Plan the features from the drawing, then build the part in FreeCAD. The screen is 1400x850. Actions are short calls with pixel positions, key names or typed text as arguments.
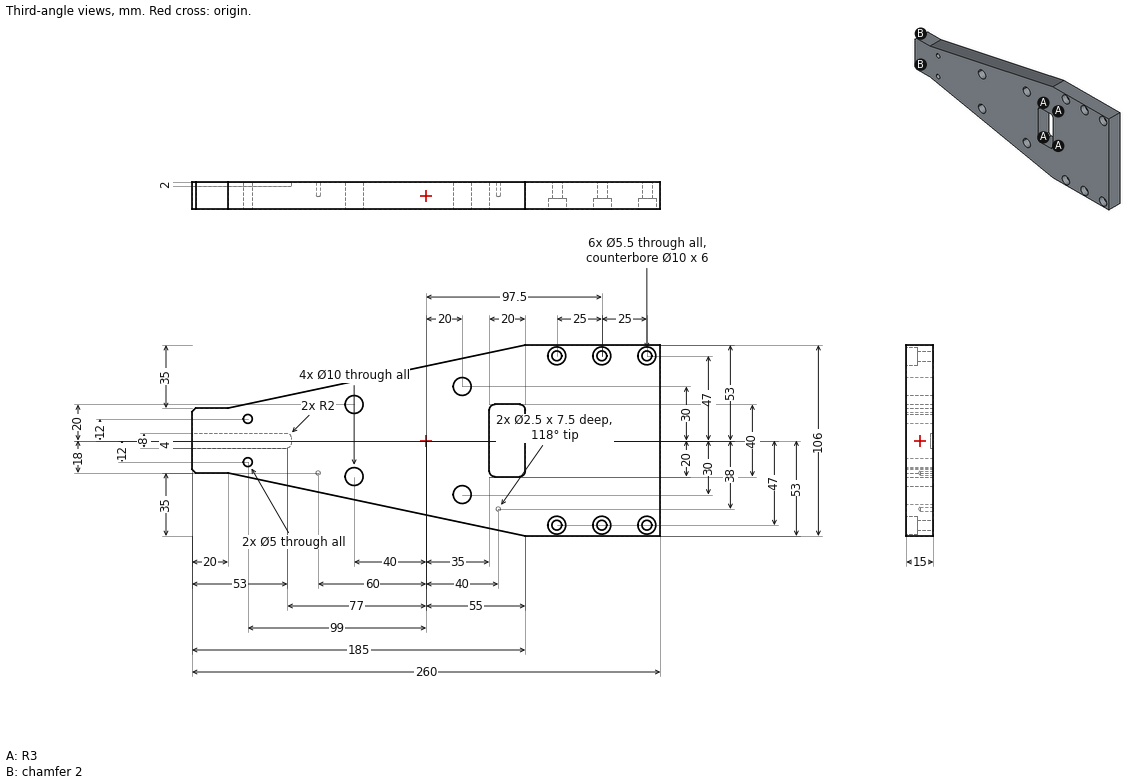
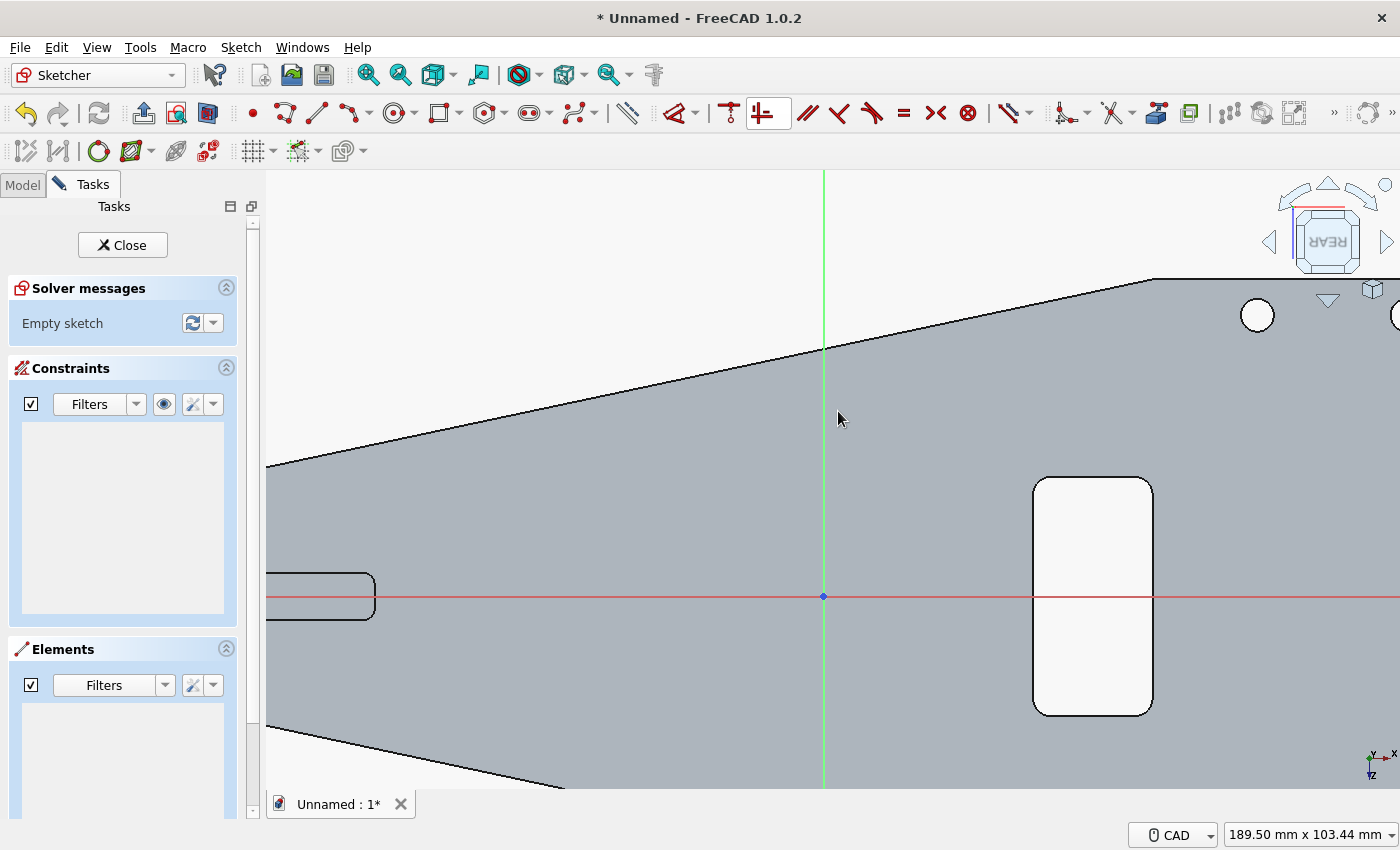
key(g)
key(c)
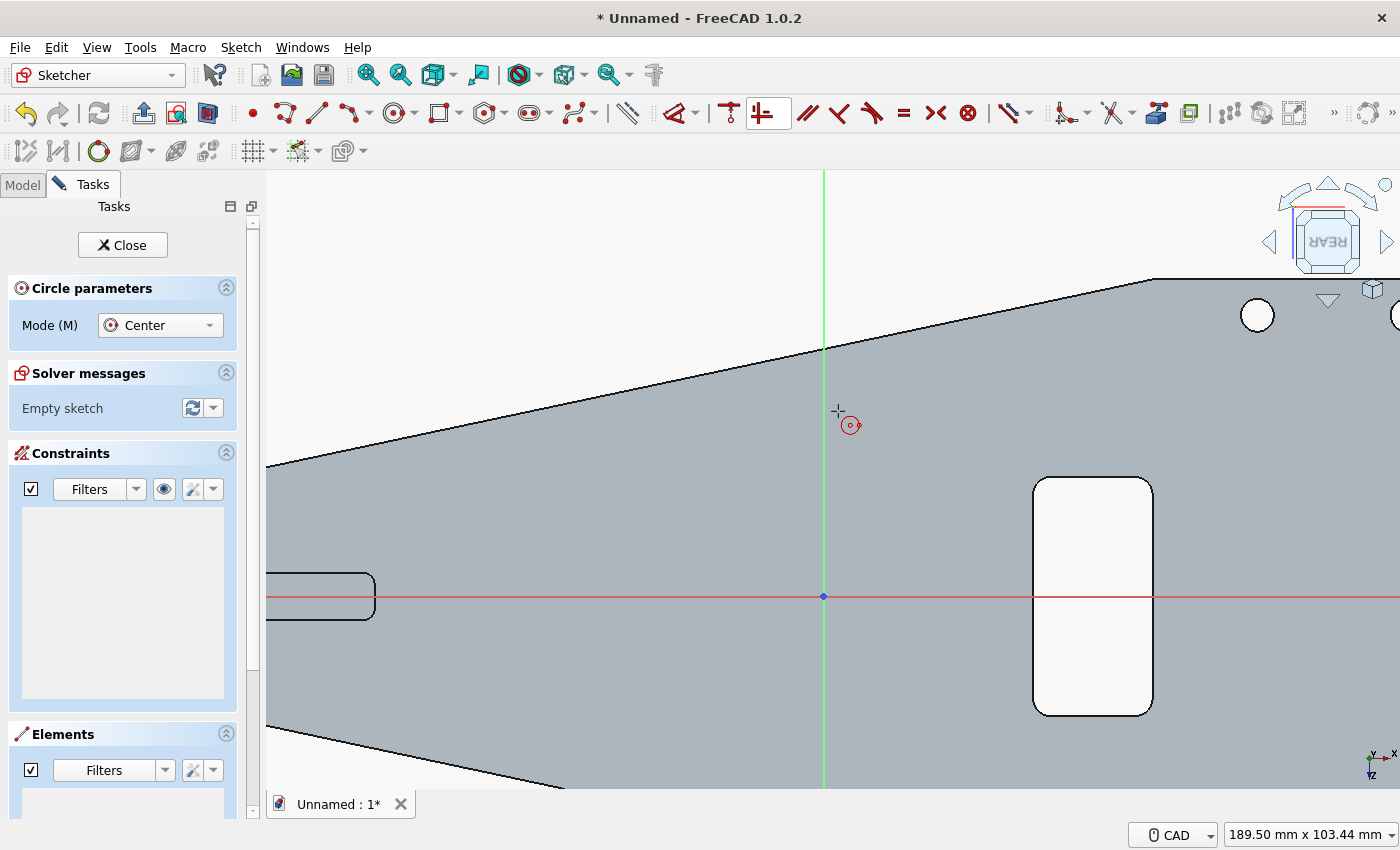
scroll(1063, 369, up, 6)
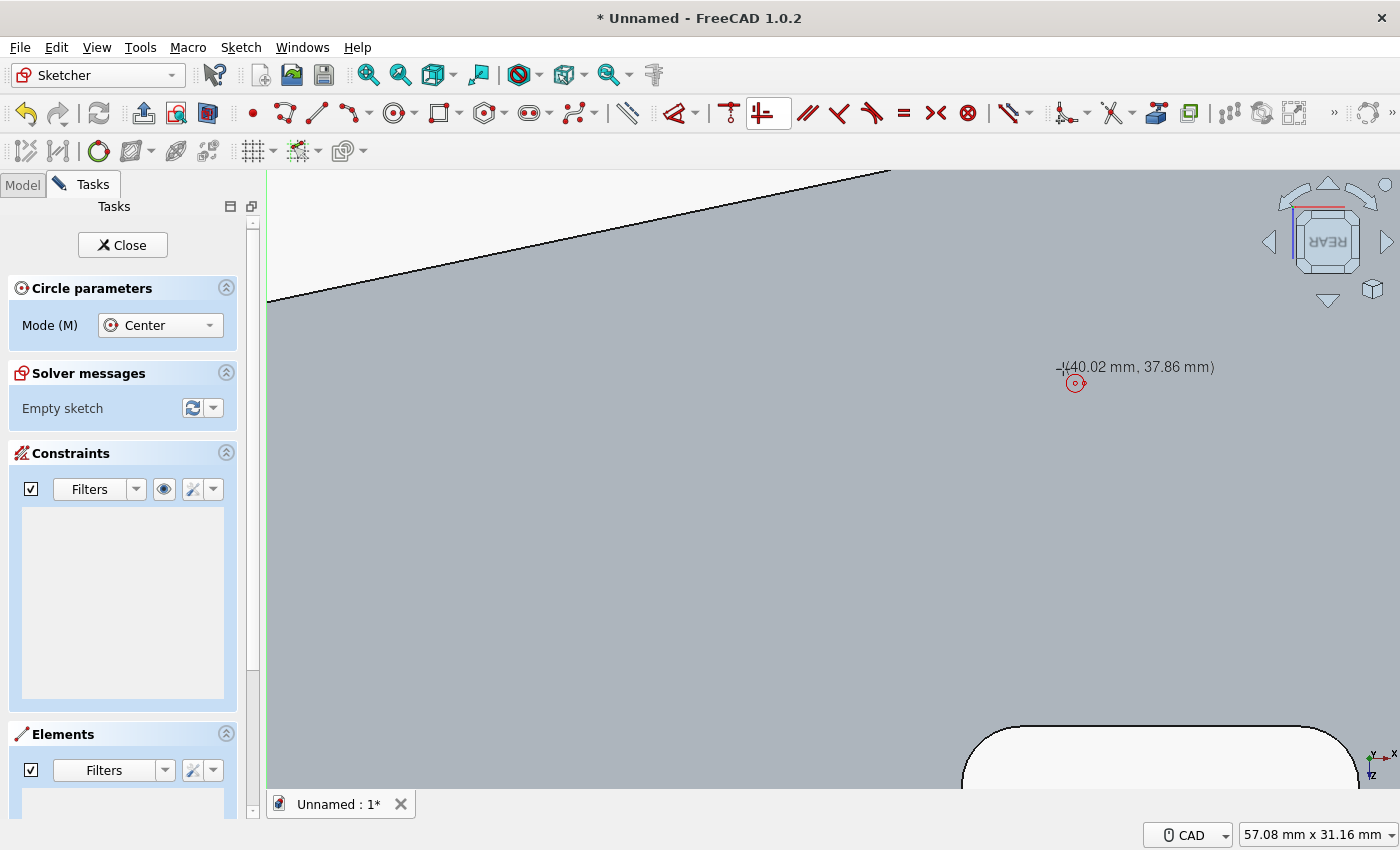
click(1061, 369)
click(1079, 351)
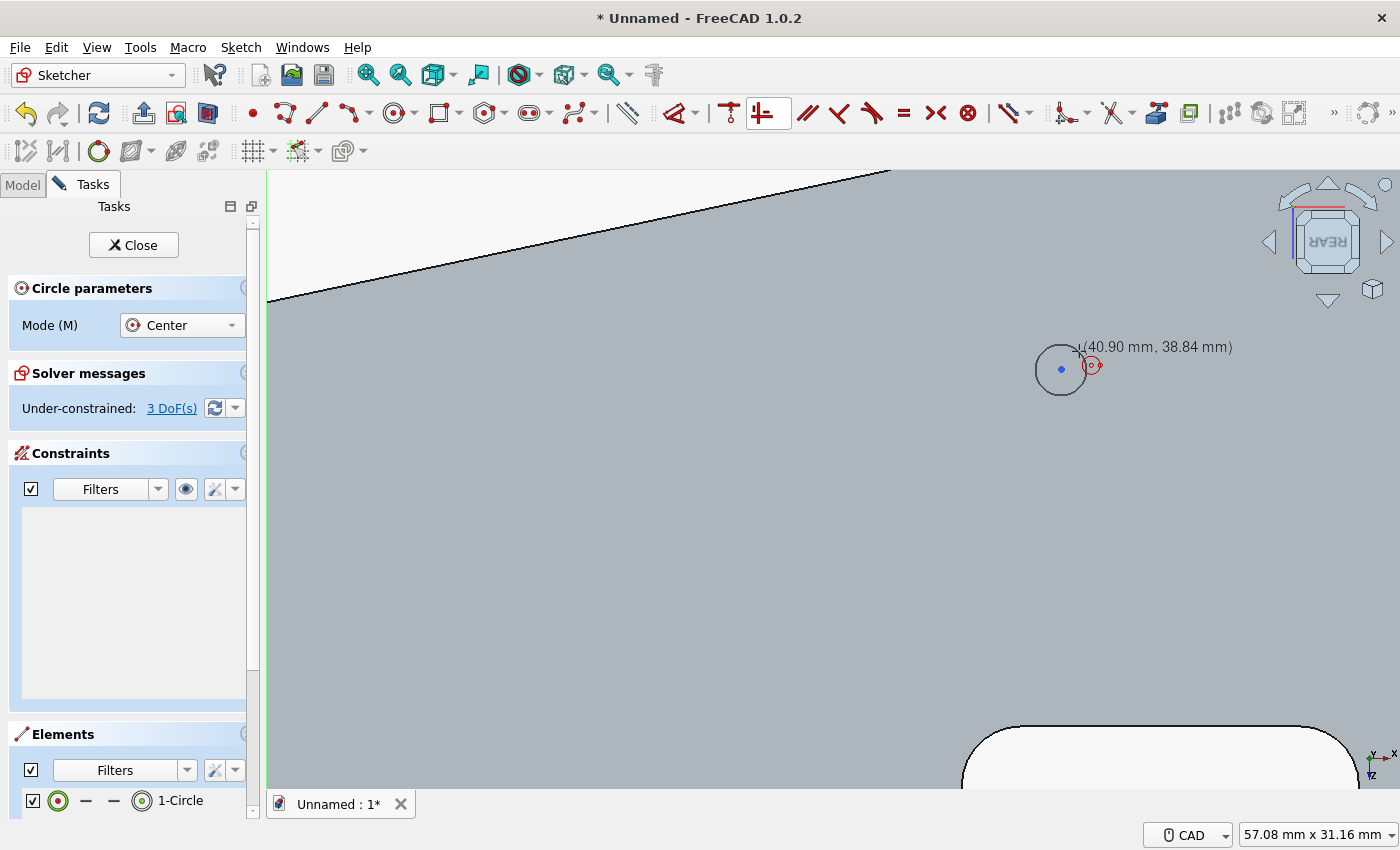
scroll(1065, 370, down, 6)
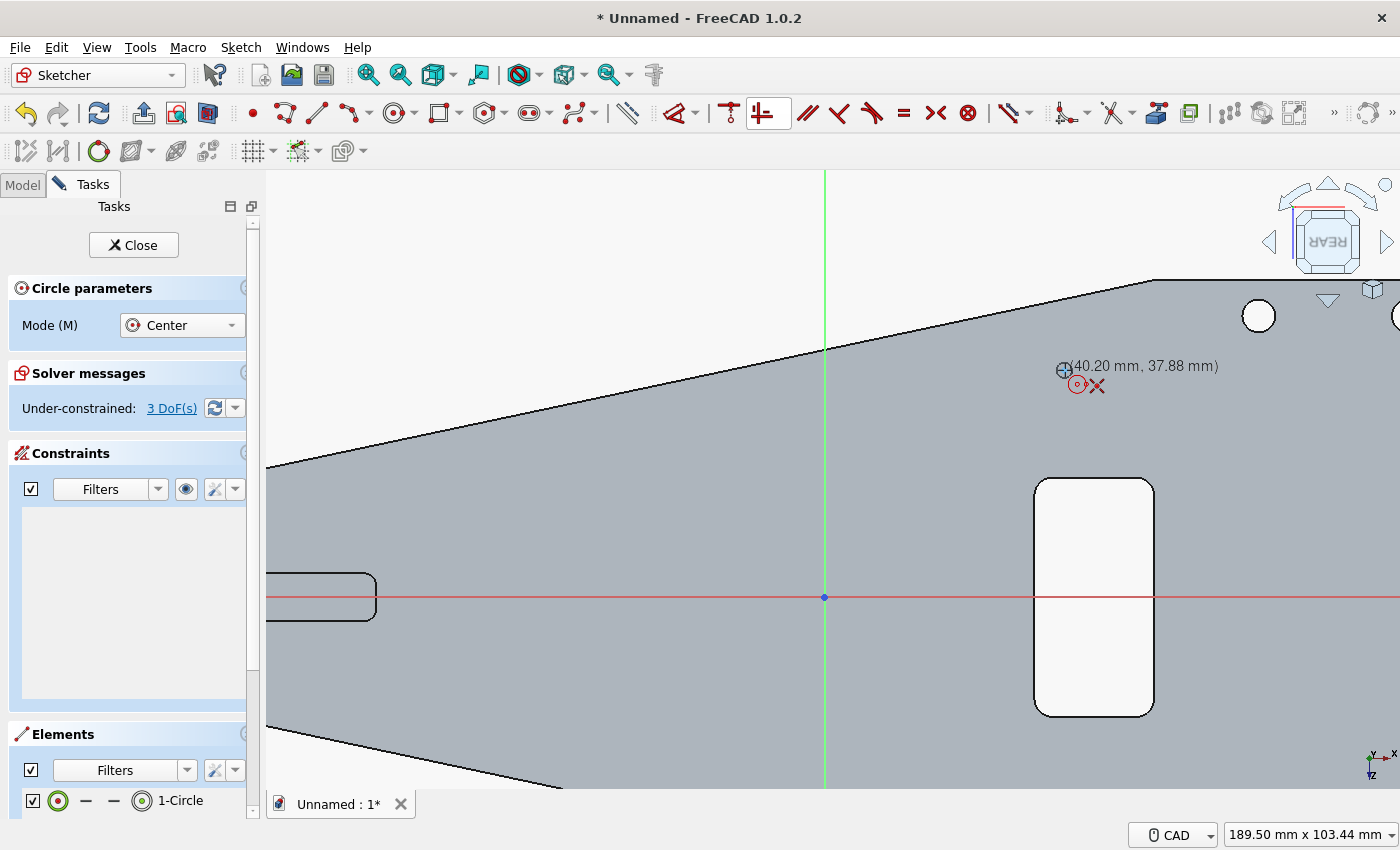
scroll(466, 490, up, 6)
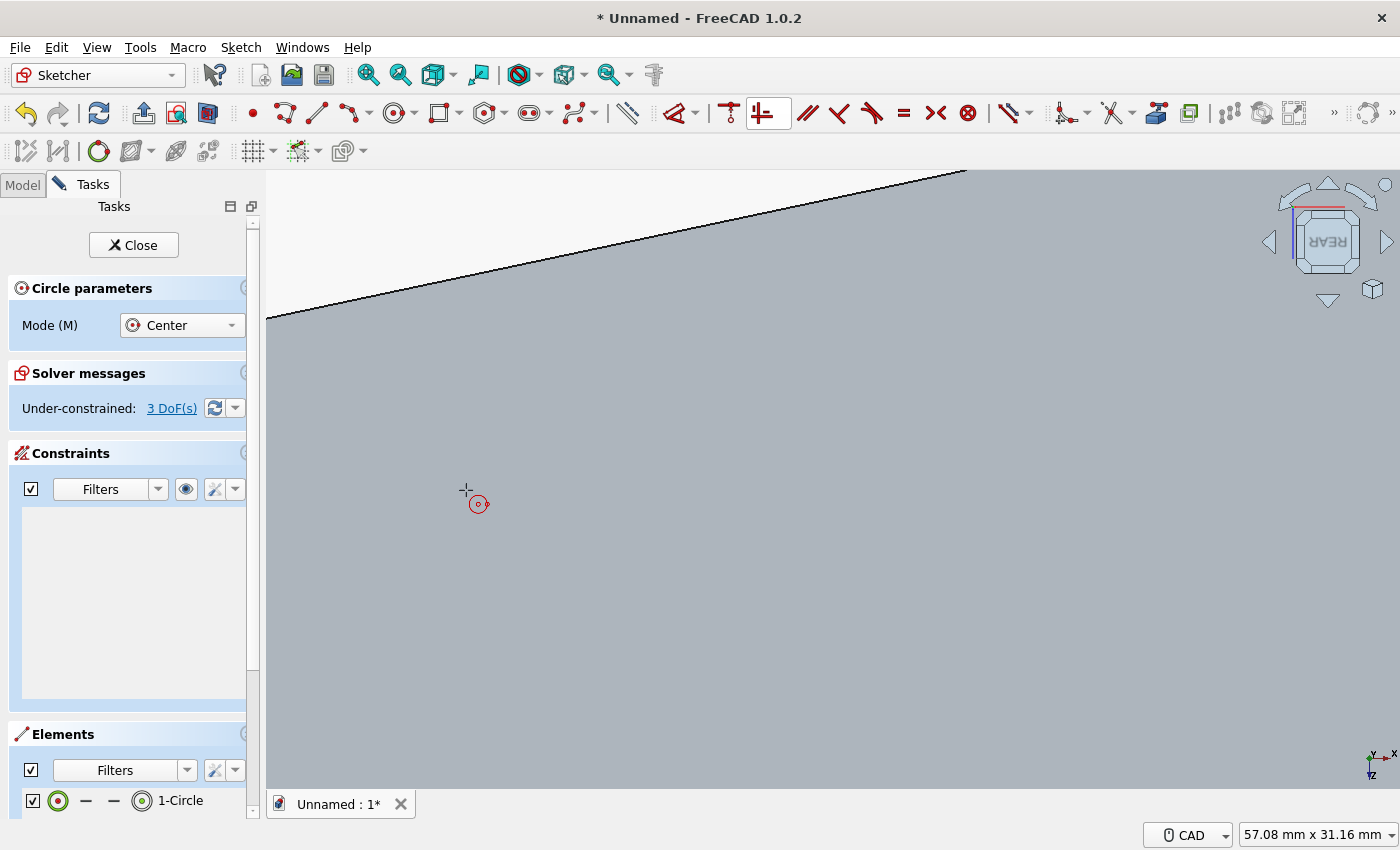
click(465, 487)
click(483, 470)
key(Escape)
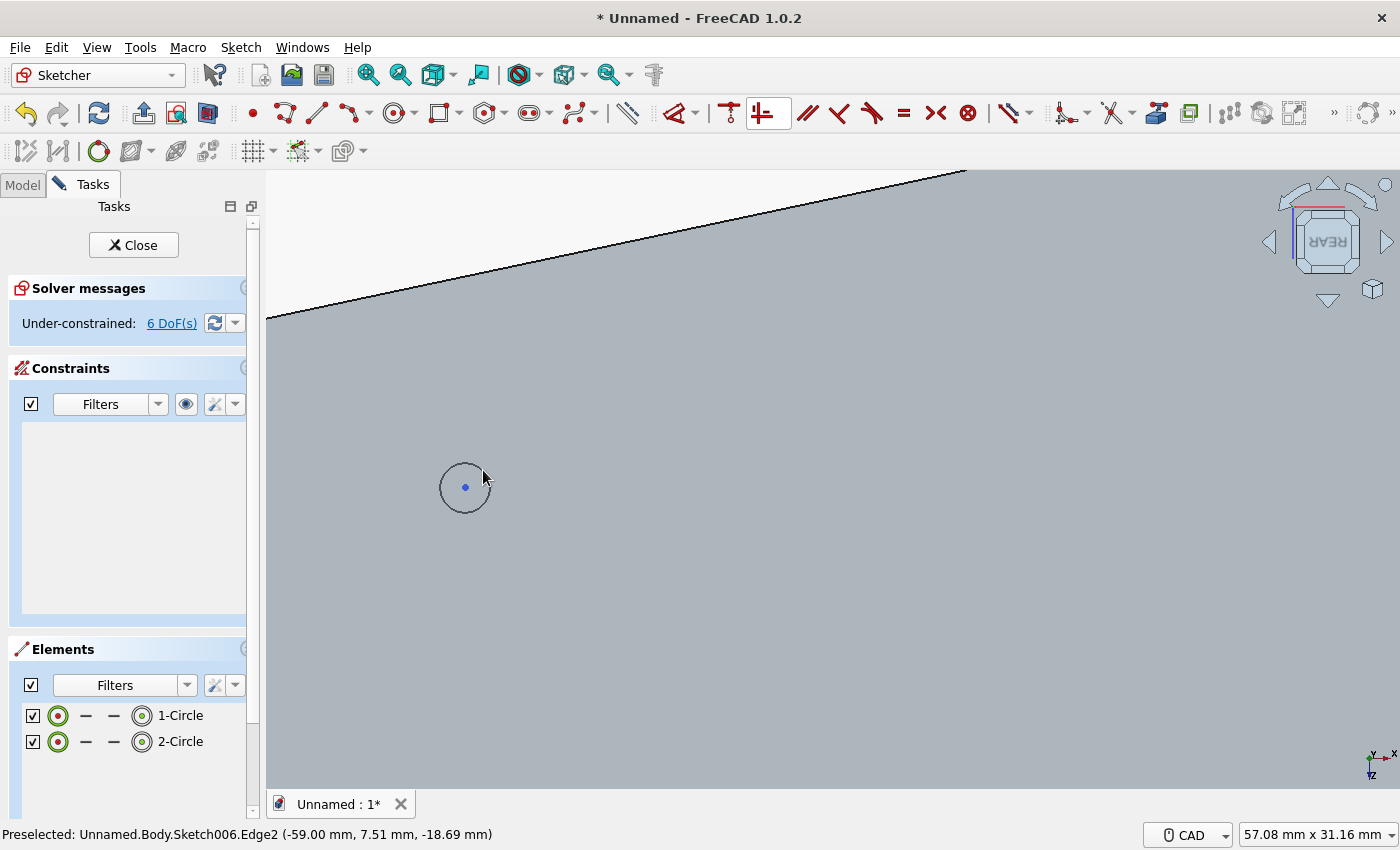
scroll(465, 490, down, 6)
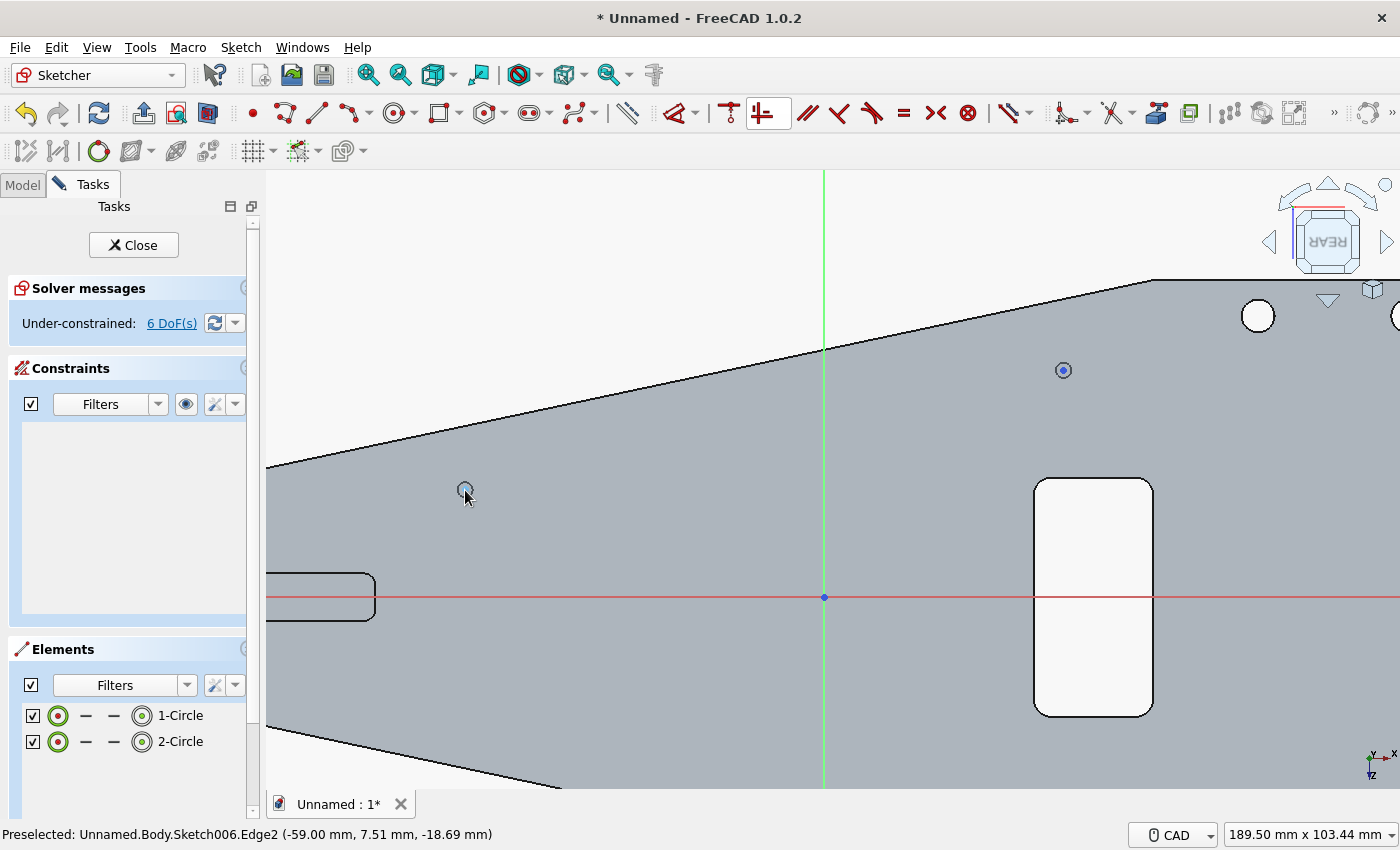
scroll(1069, 365, up, 3)